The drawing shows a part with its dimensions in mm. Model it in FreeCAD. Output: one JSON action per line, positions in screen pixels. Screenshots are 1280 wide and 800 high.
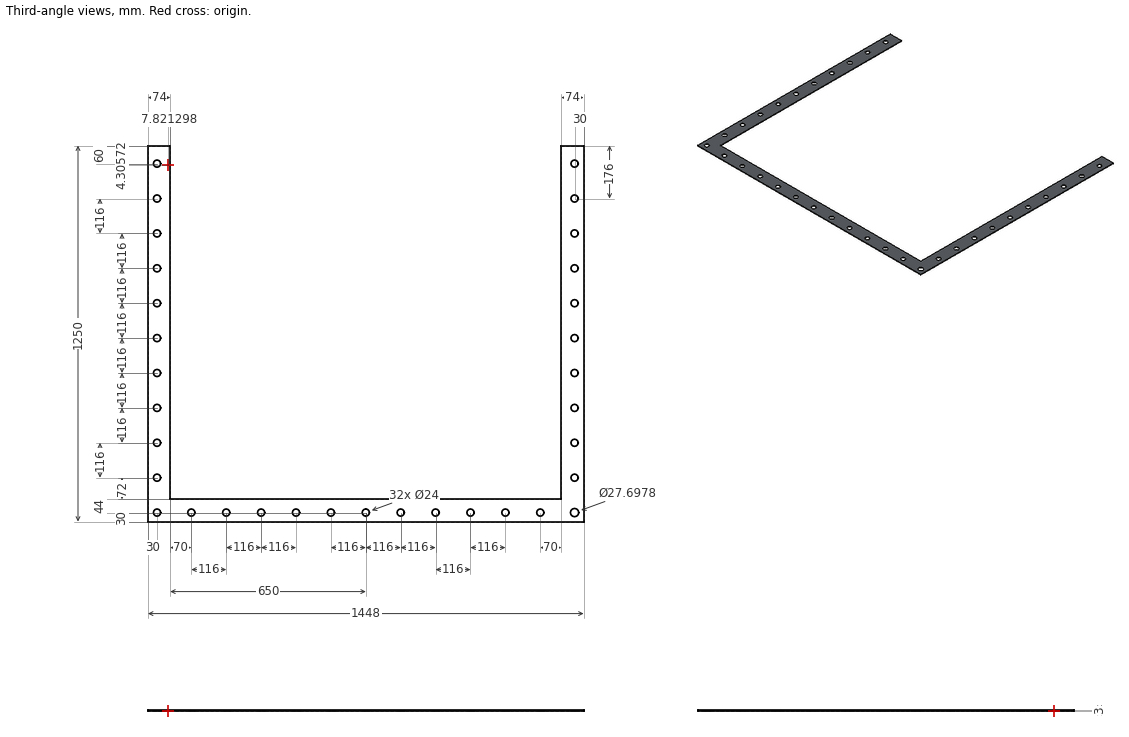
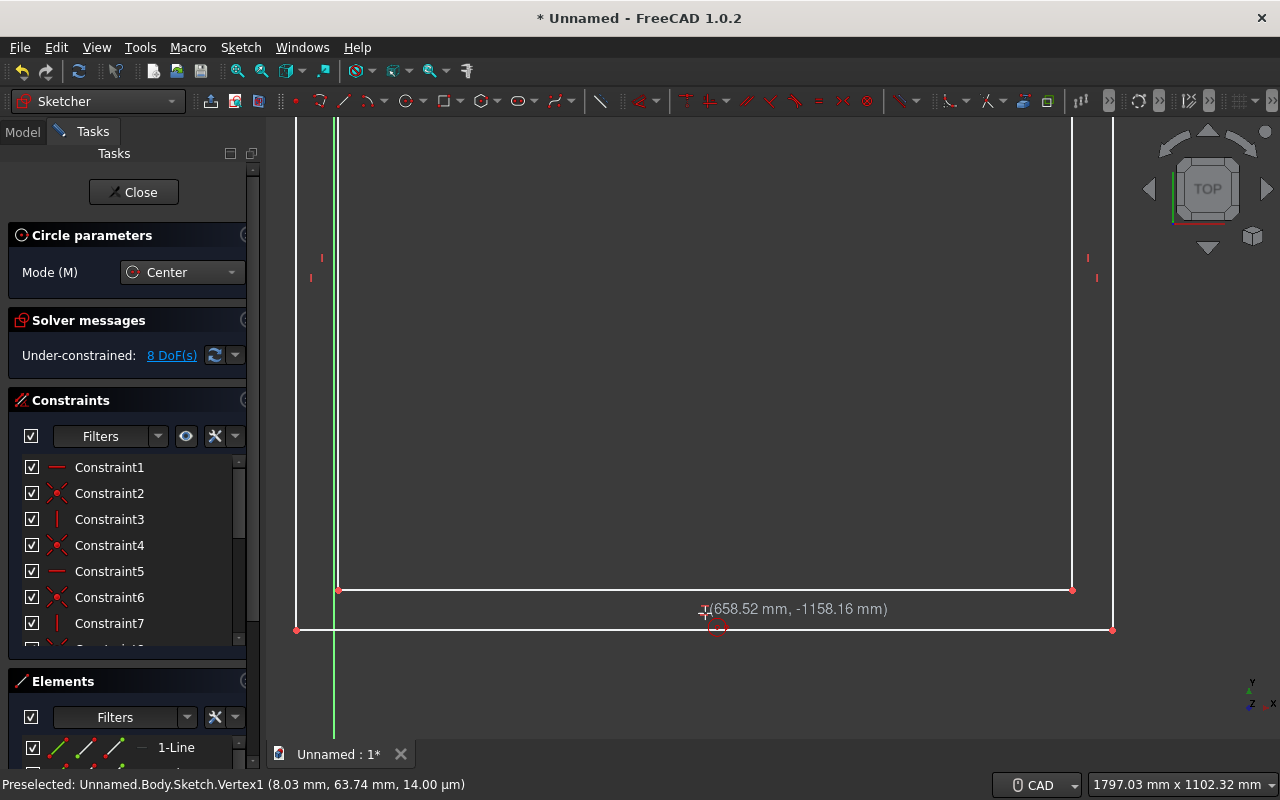
{"action": "left_click", "coordinate": [705, 612]}
{"action": "mouse_move", "coordinate": [710, 608]}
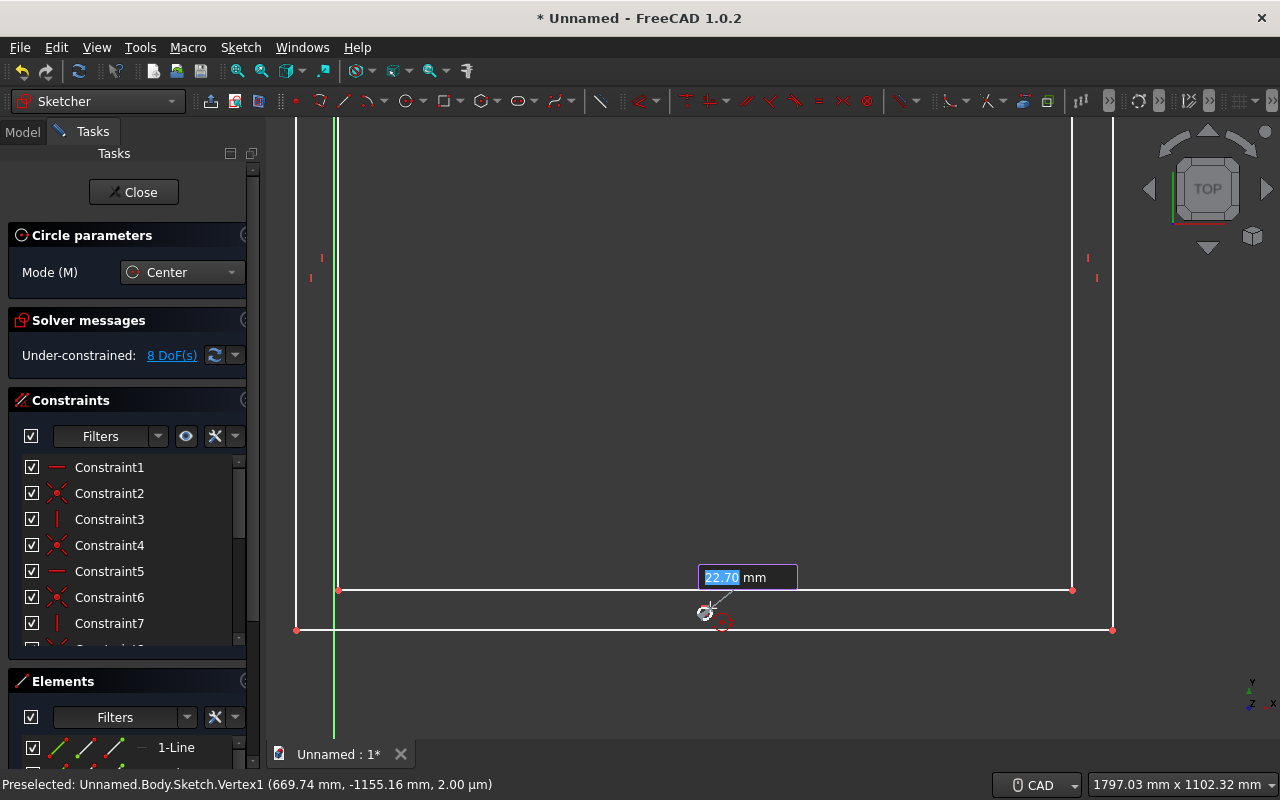
{"action": "type", "text": "24"}
{"action": "key", "text": "Return"}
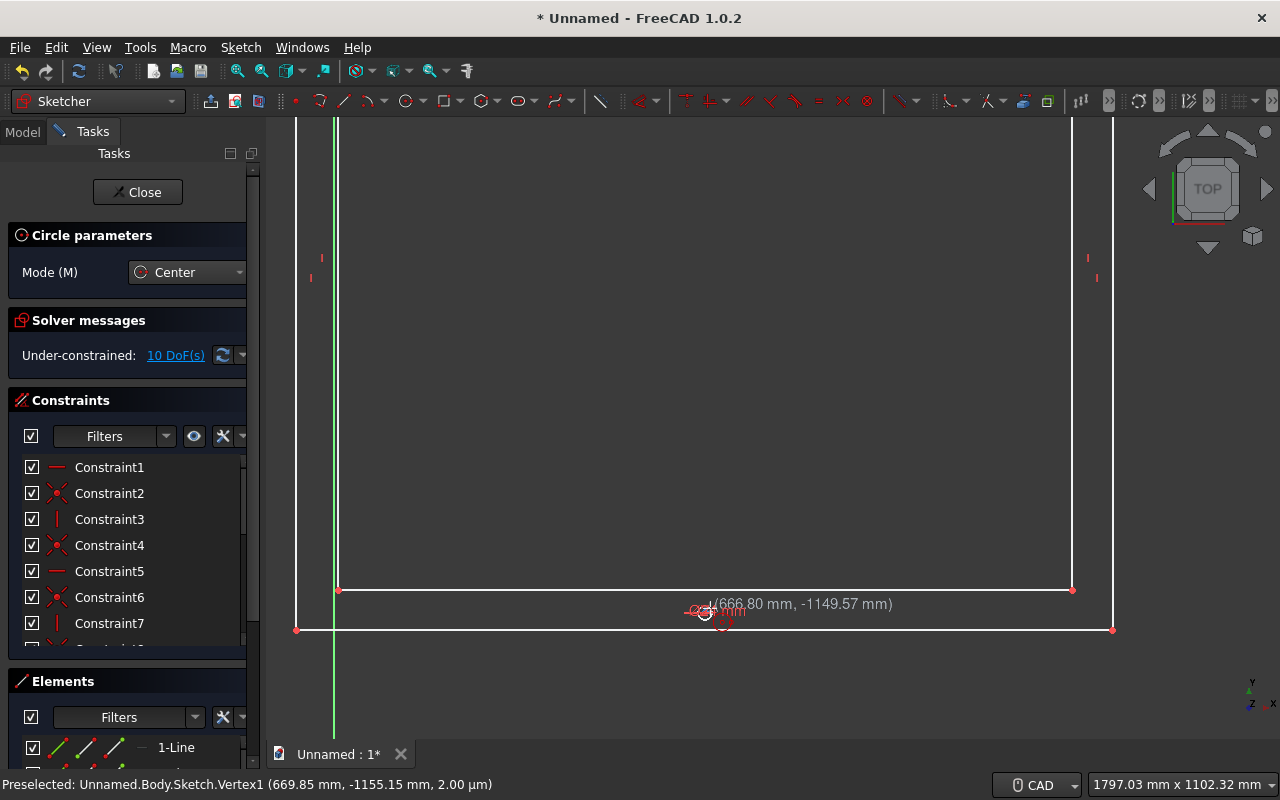
{"action": "scroll", "coordinate": [313, 612], "scroll_direction": "up", "scroll_amount": 7}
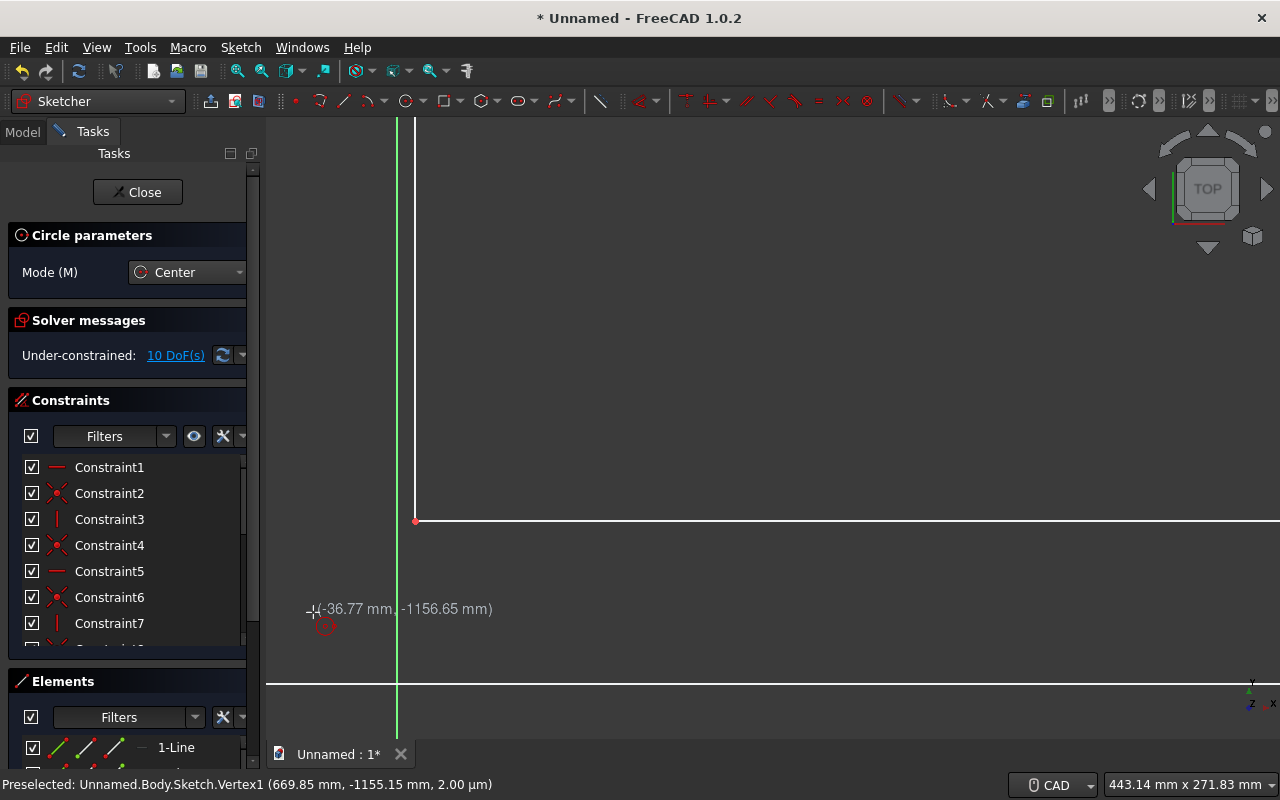
{"action": "scroll", "coordinate": [517, 612], "scroll_direction": "down", "scroll_amount": 10}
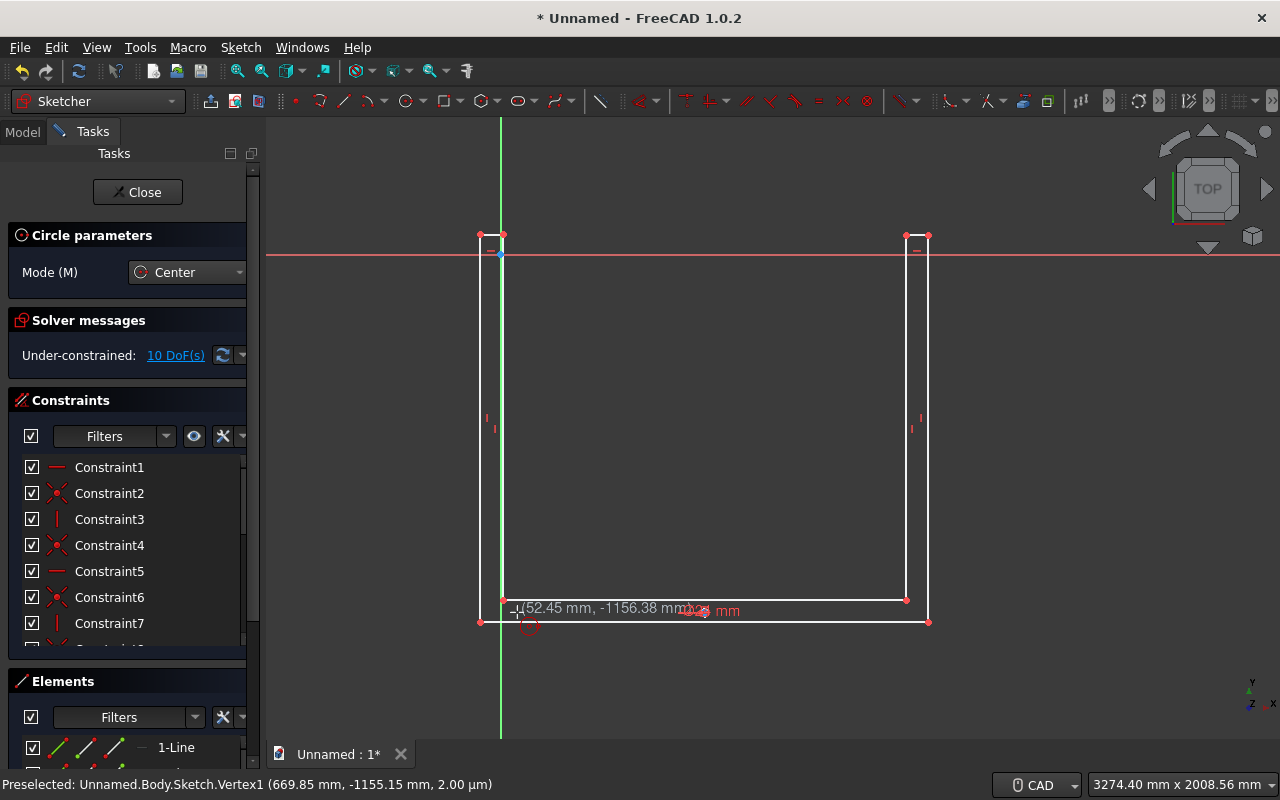
{"action": "scroll", "coordinate": [490, 613], "scroll_direction": "up", "scroll_amount": 3}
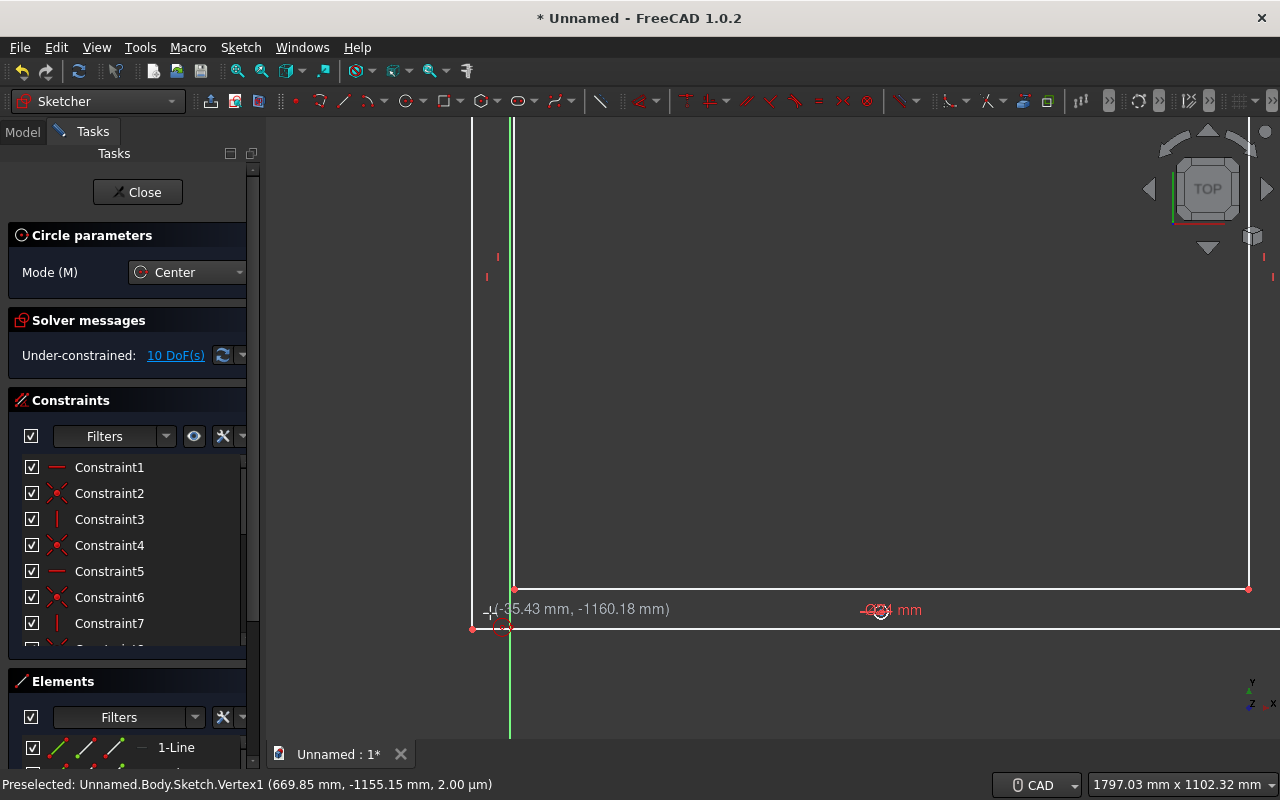
{"action": "left_click", "coordinate": [489, 612]}
{"action": "mouse_move", "coordinate": [494, 607]}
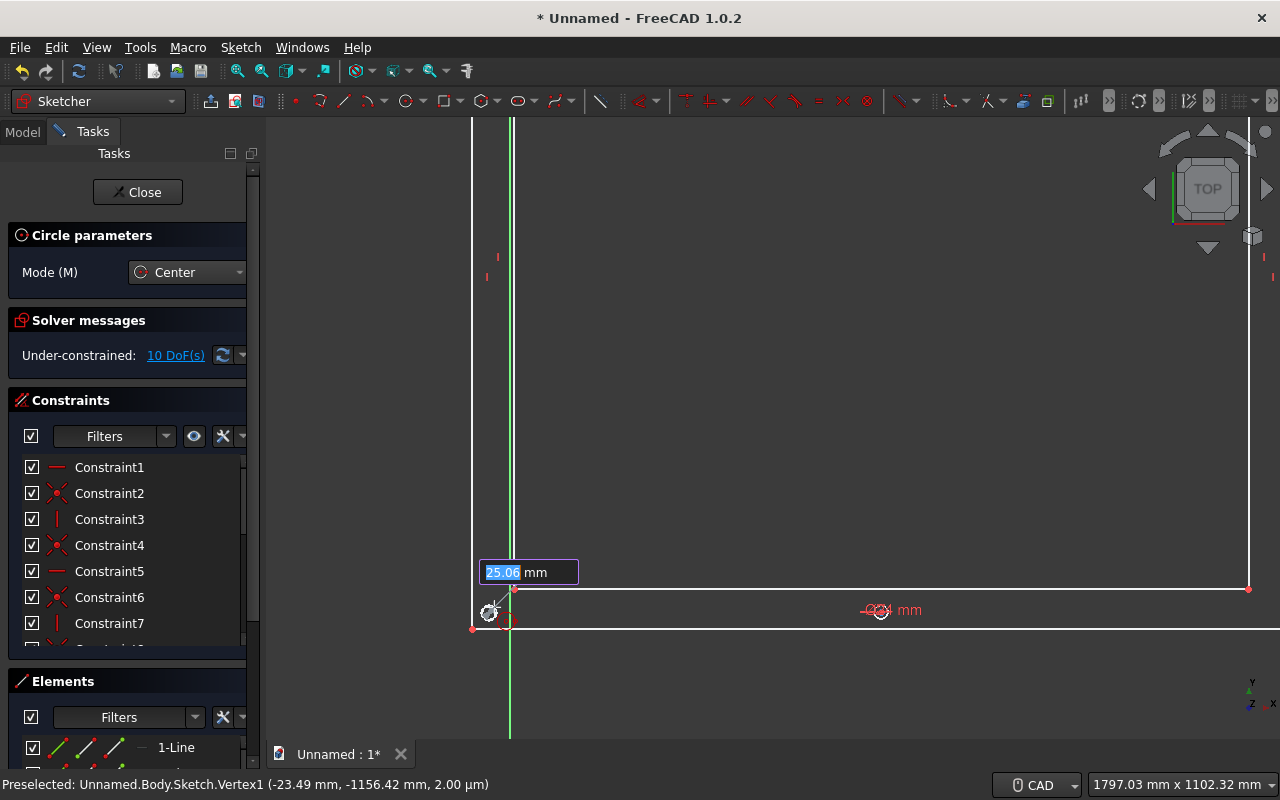
{"action": "type", "text": "24"}
{"action": "key", "text": "Return"}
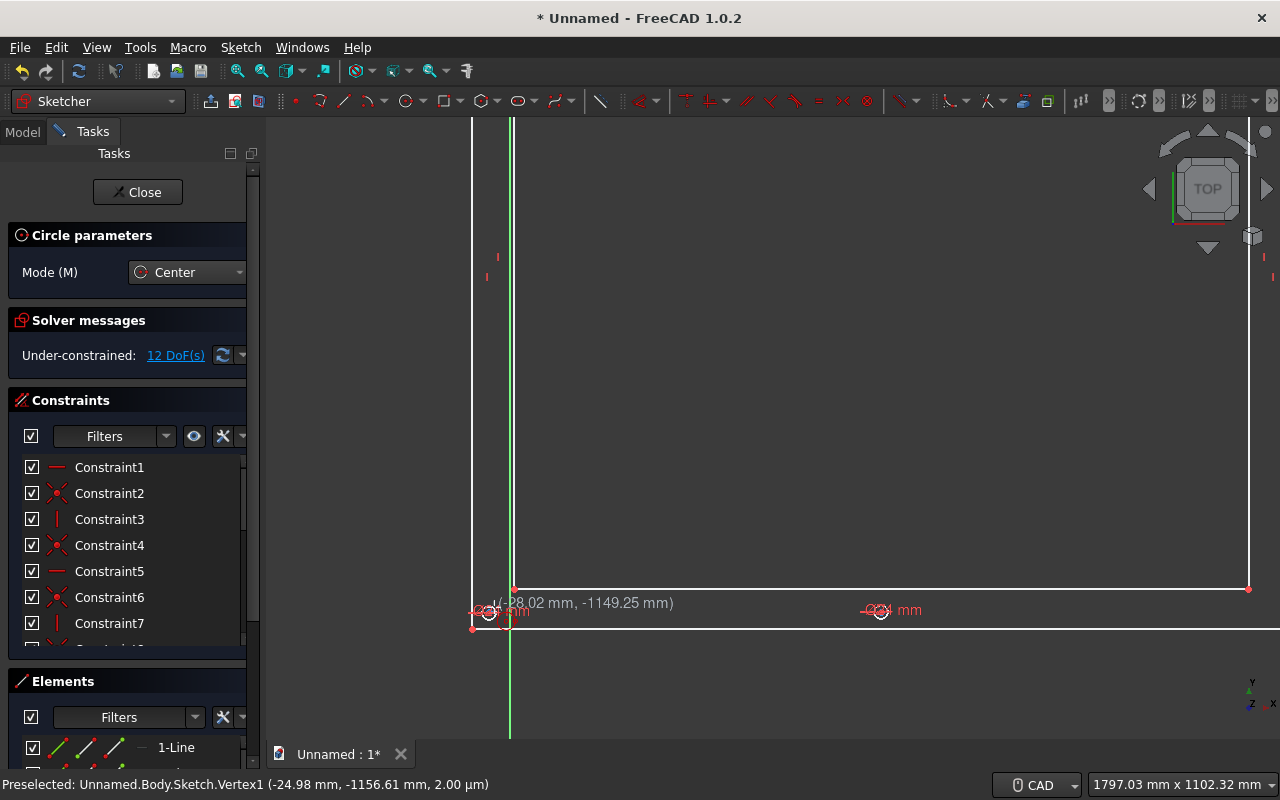
{"action": "scroll", "coordinate": [489, 546], "scroll_direction": "up", "scroll_amount": 7}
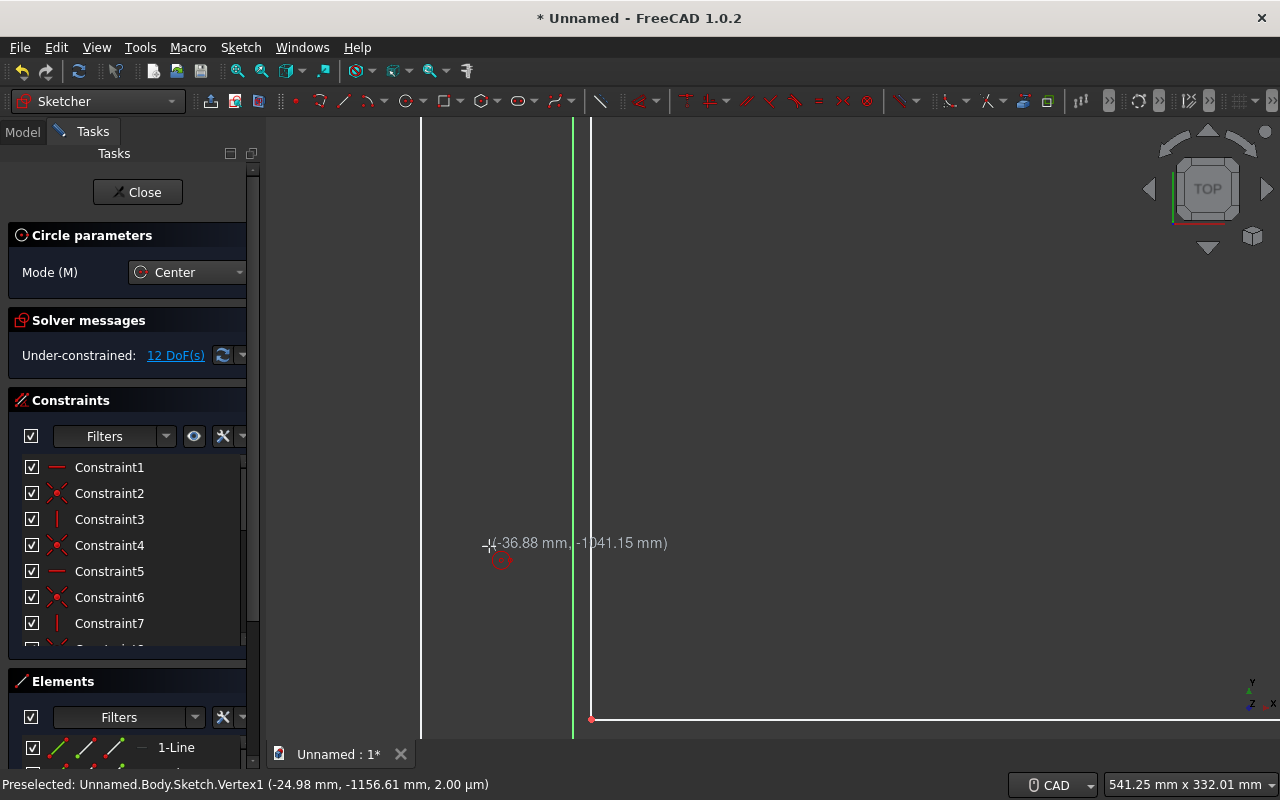
{"action": "scroll", "coordinate": [490, 581], "scroll_direction": "down", "scroll_amount": 10}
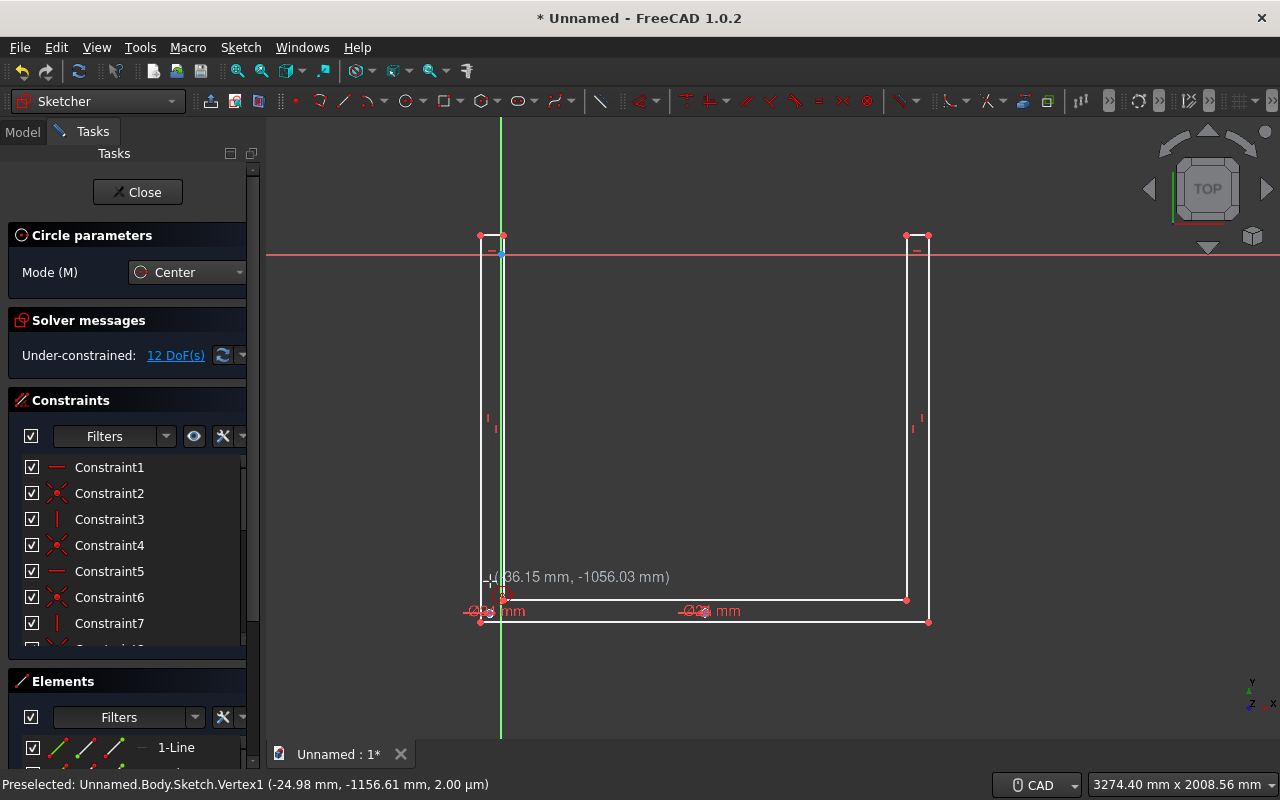
{"action": "scroll", "coordinate": [490, 577], "scroll_direction": "up", "scroll_amount": 3}